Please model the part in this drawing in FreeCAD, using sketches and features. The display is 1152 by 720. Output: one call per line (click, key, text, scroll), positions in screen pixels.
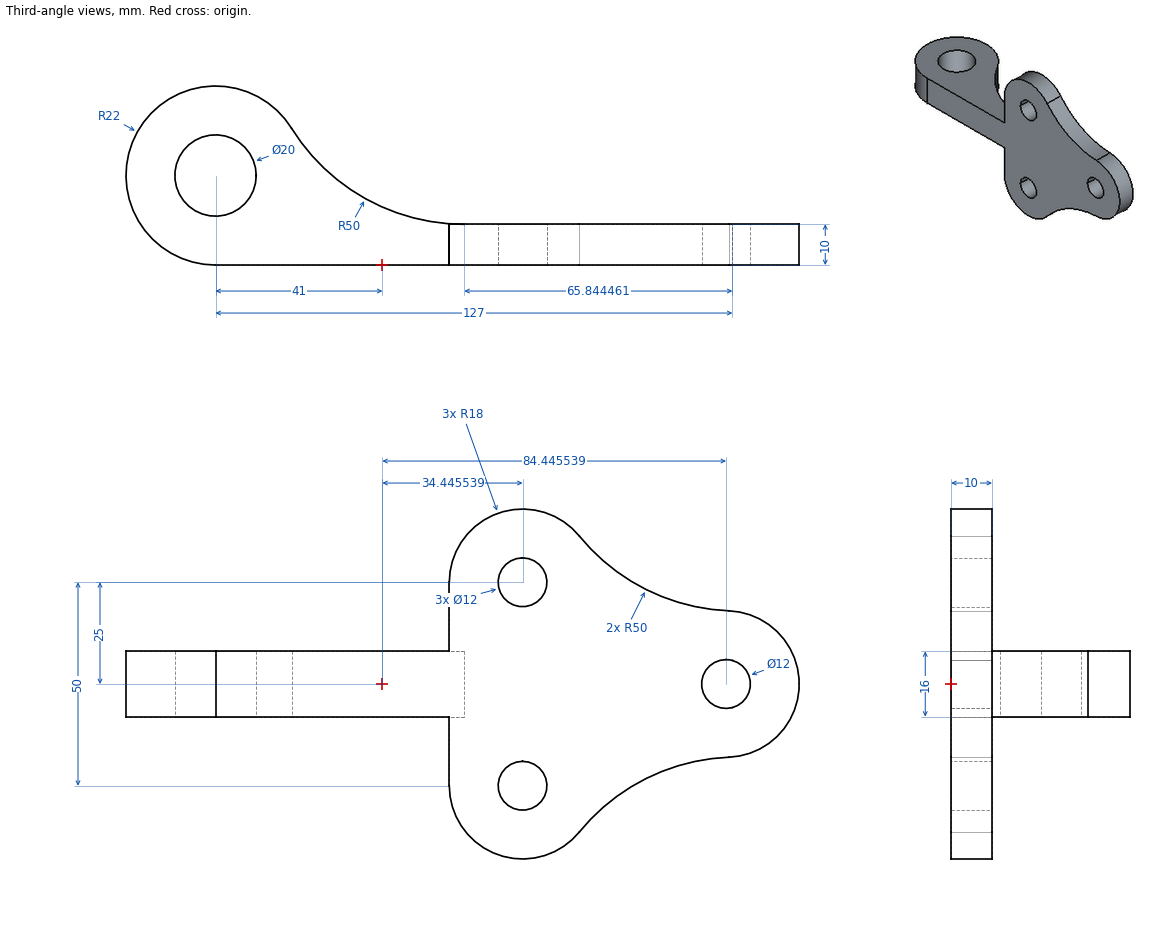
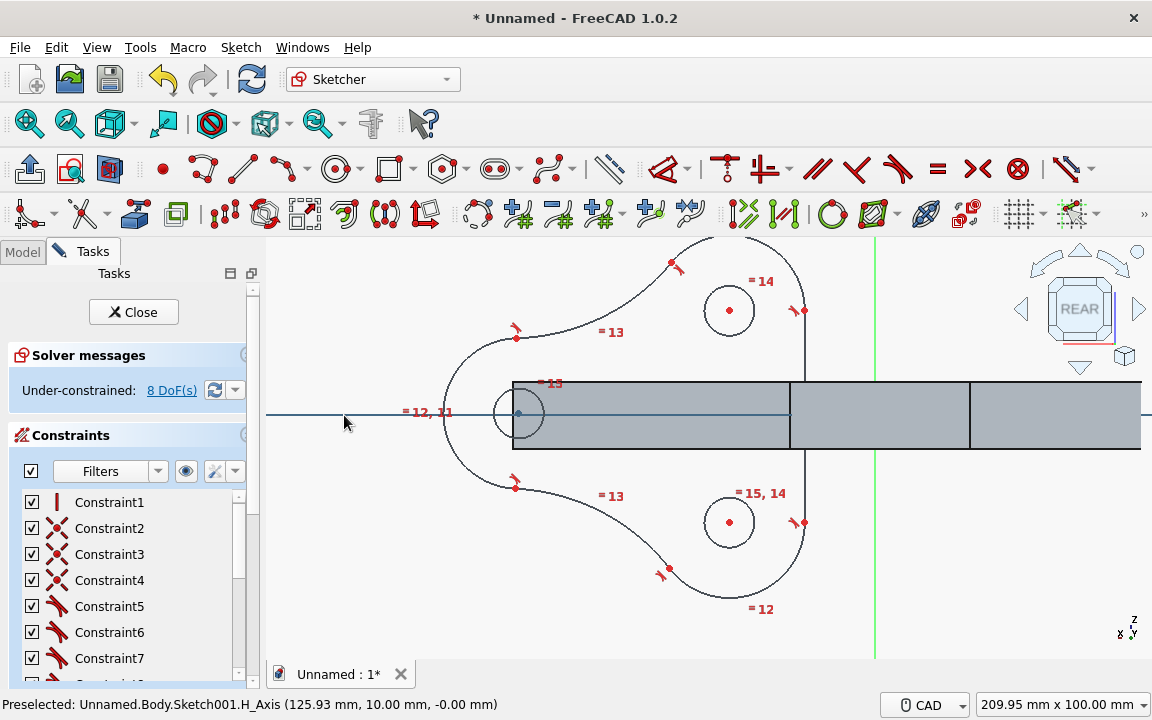
click(726, 170)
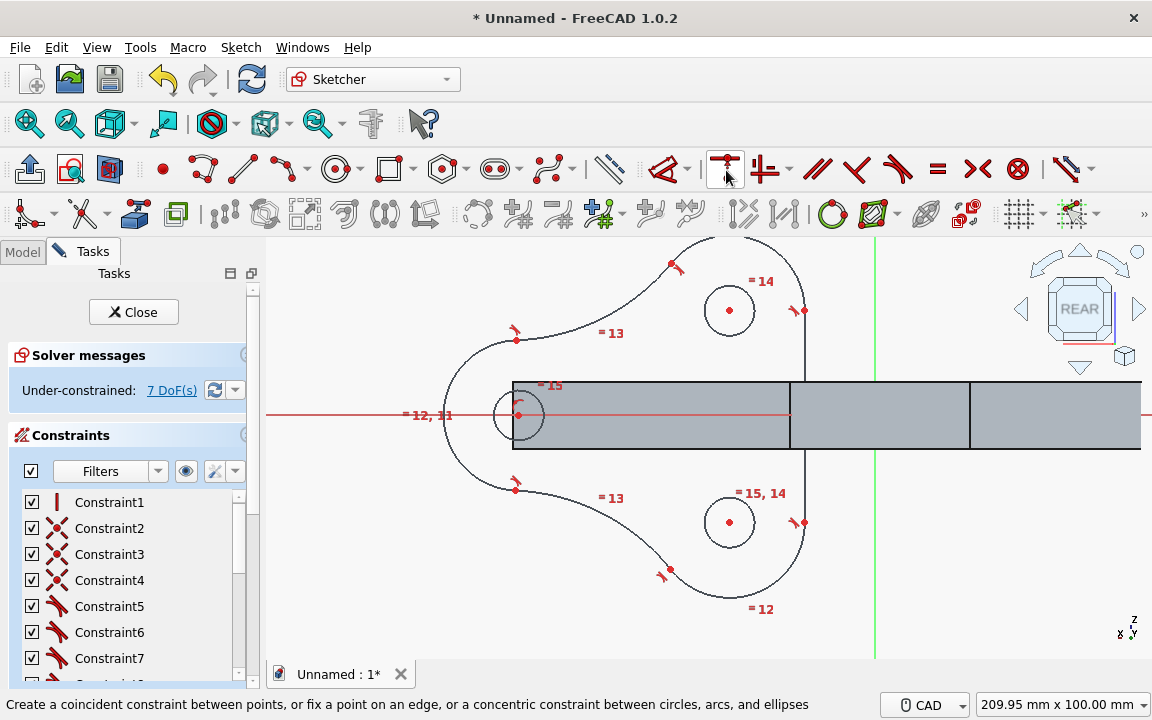
key(d)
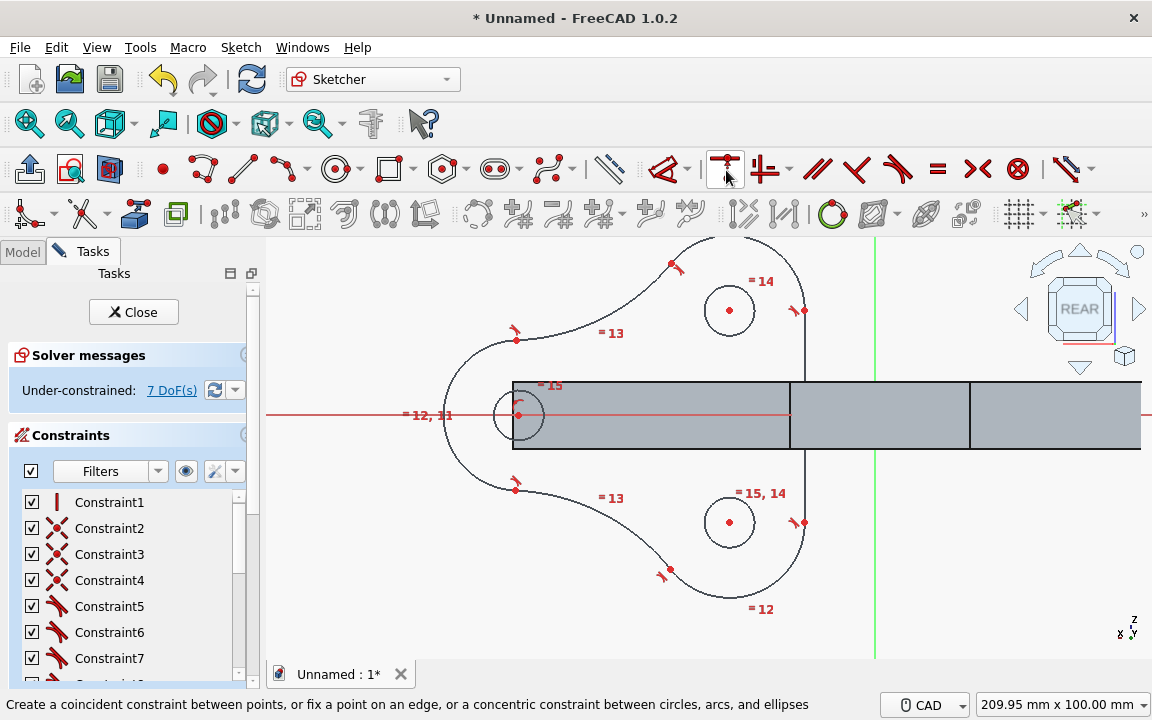
click(796, 275)
click(837, 311)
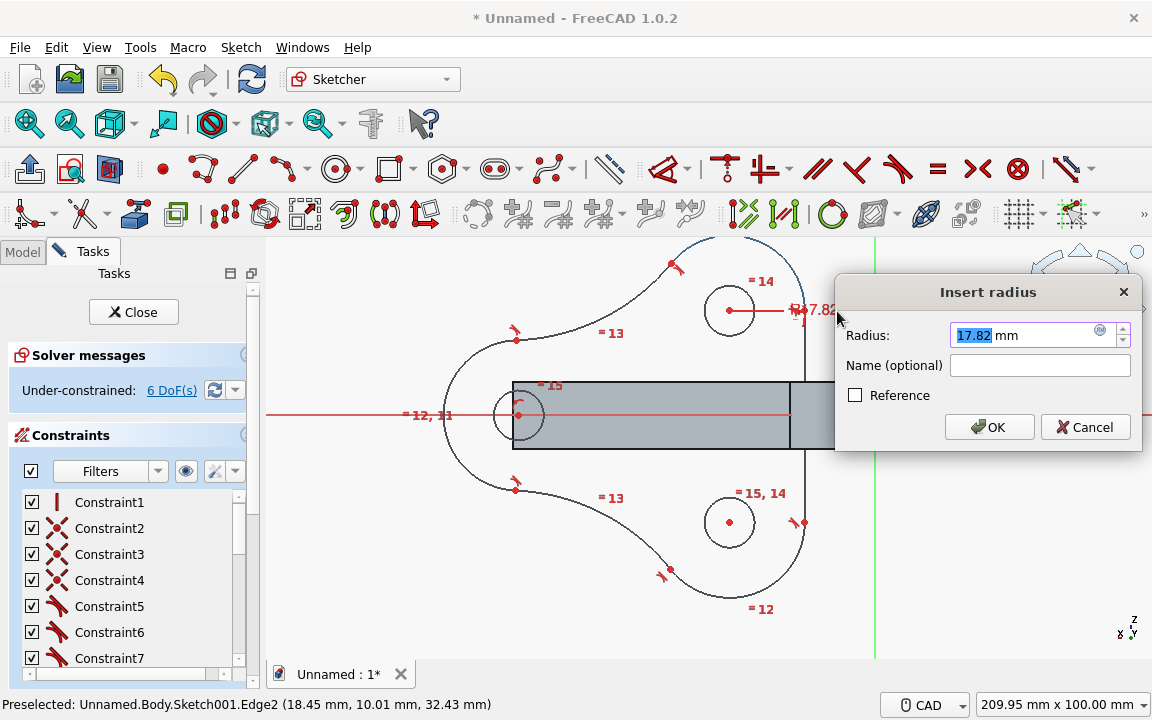
text(18)
key(Return)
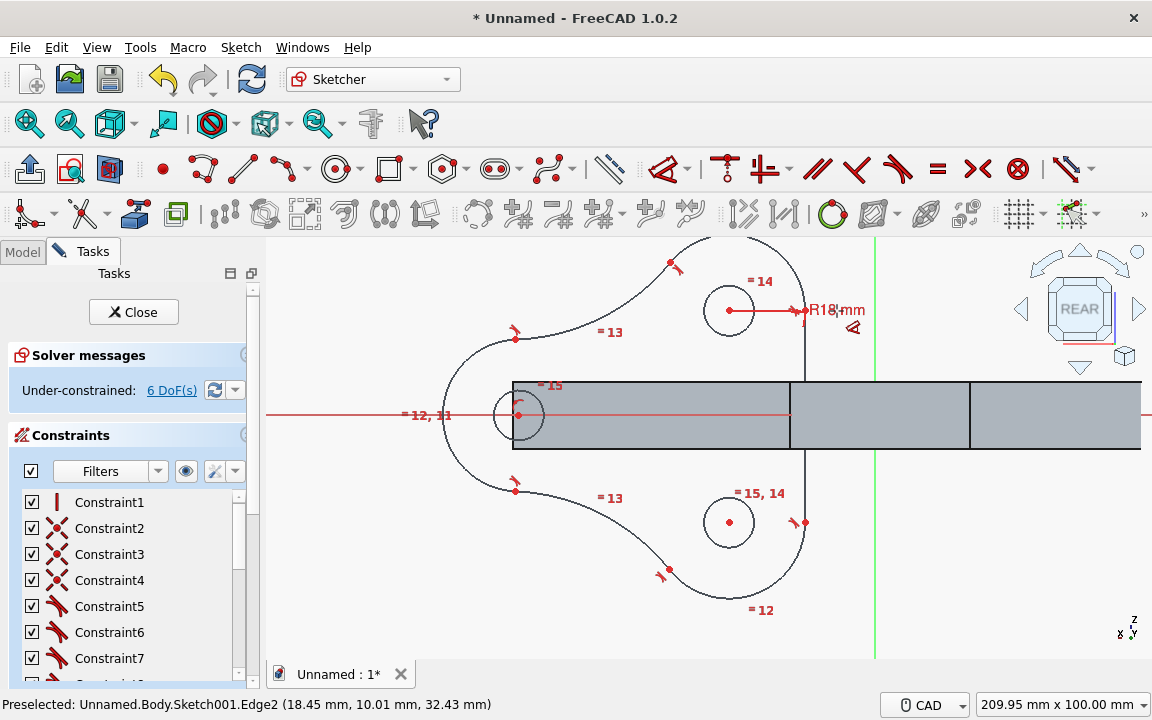
click(568, 331)
click(577, 362)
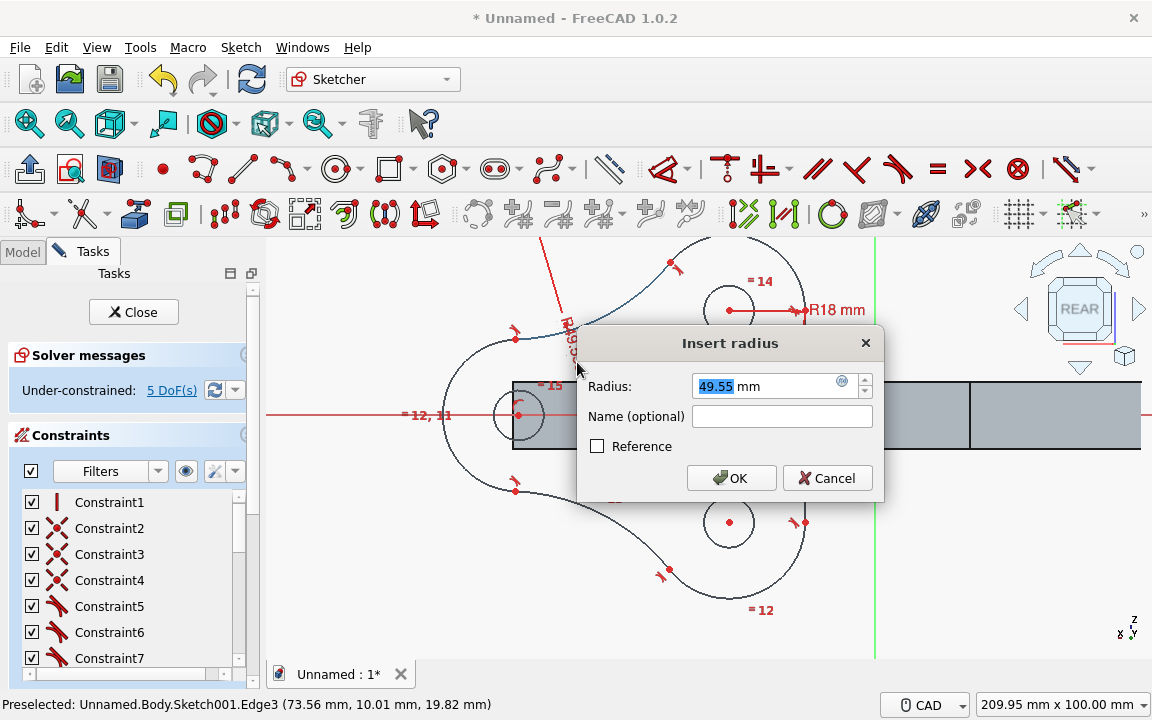
text(50)
key(Return)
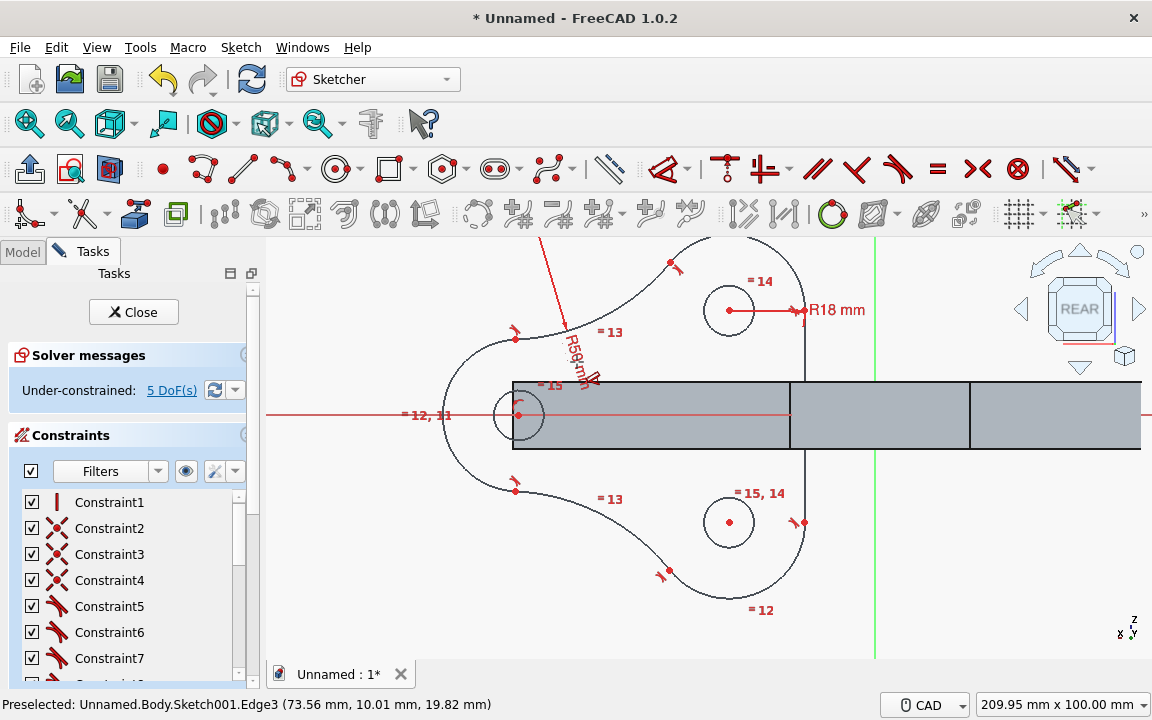
click(747, 293)
click(770, 270)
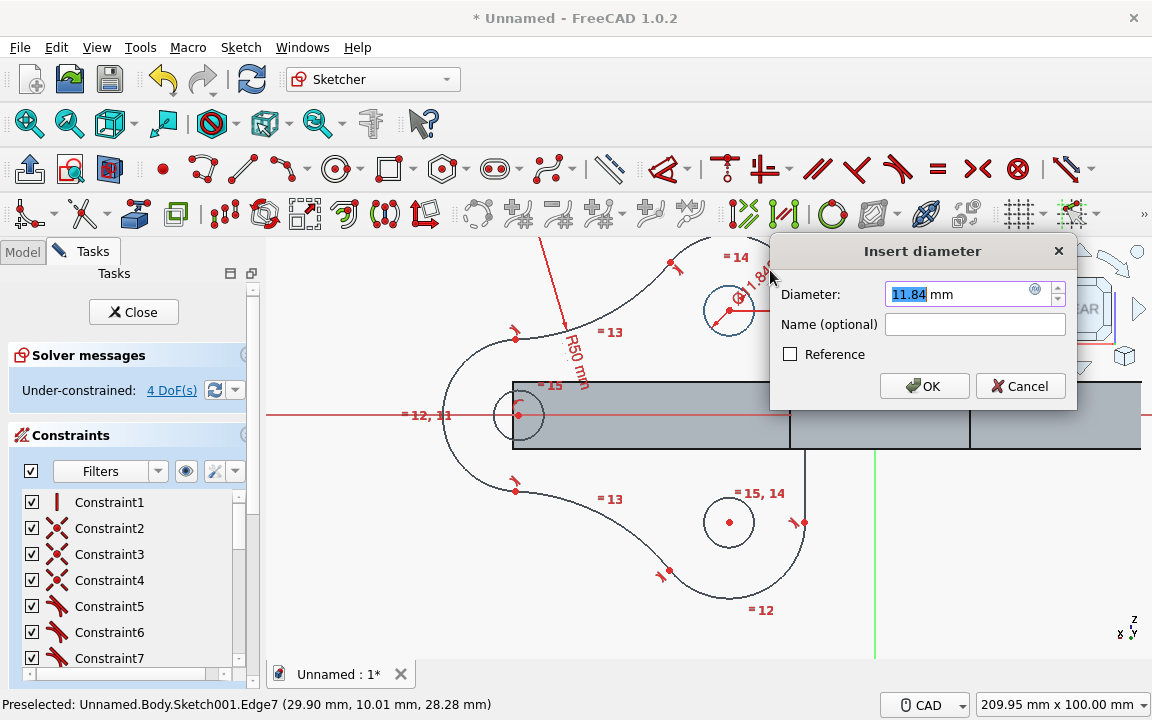
text(12)
key(Return)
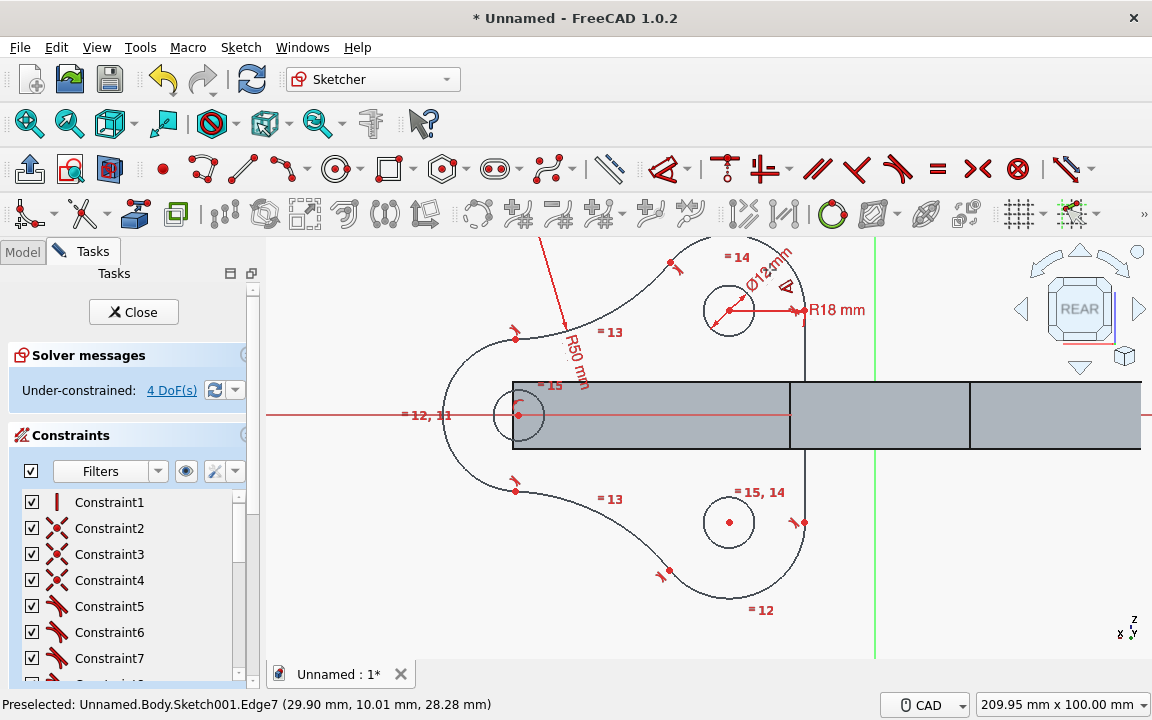
click(805, 459)
click(839, 368)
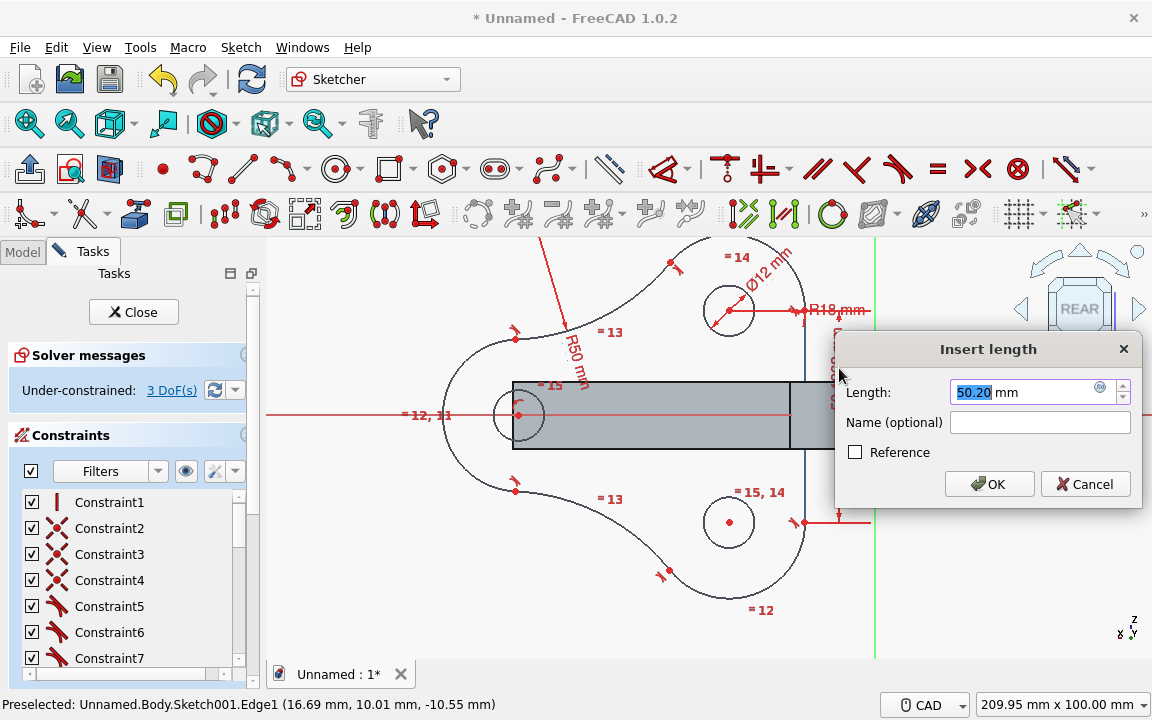
text(50)
key(Return)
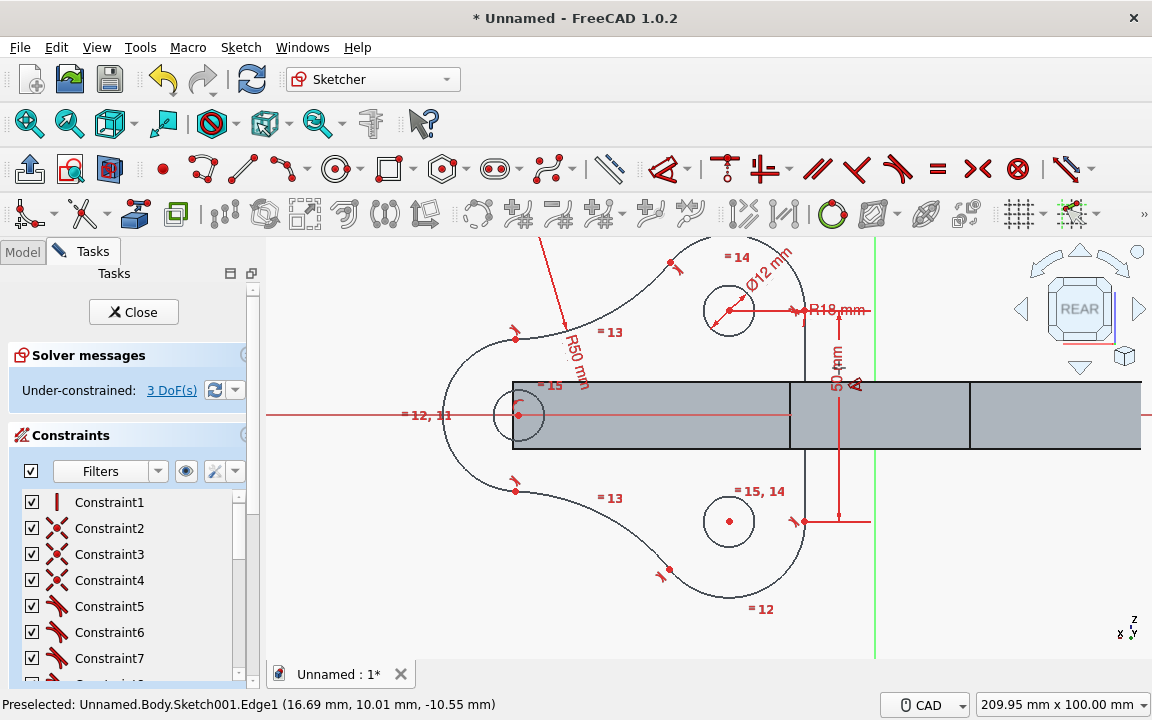
click(729, 311)
click(909, 363)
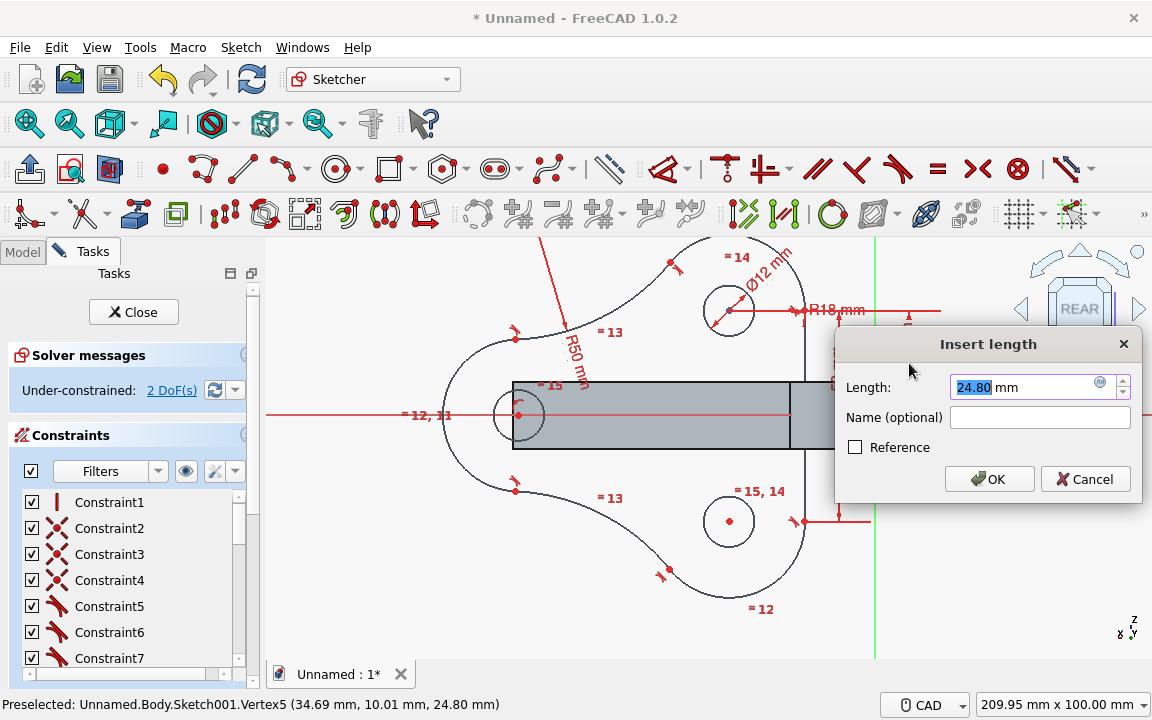
text(25)
key(Return)